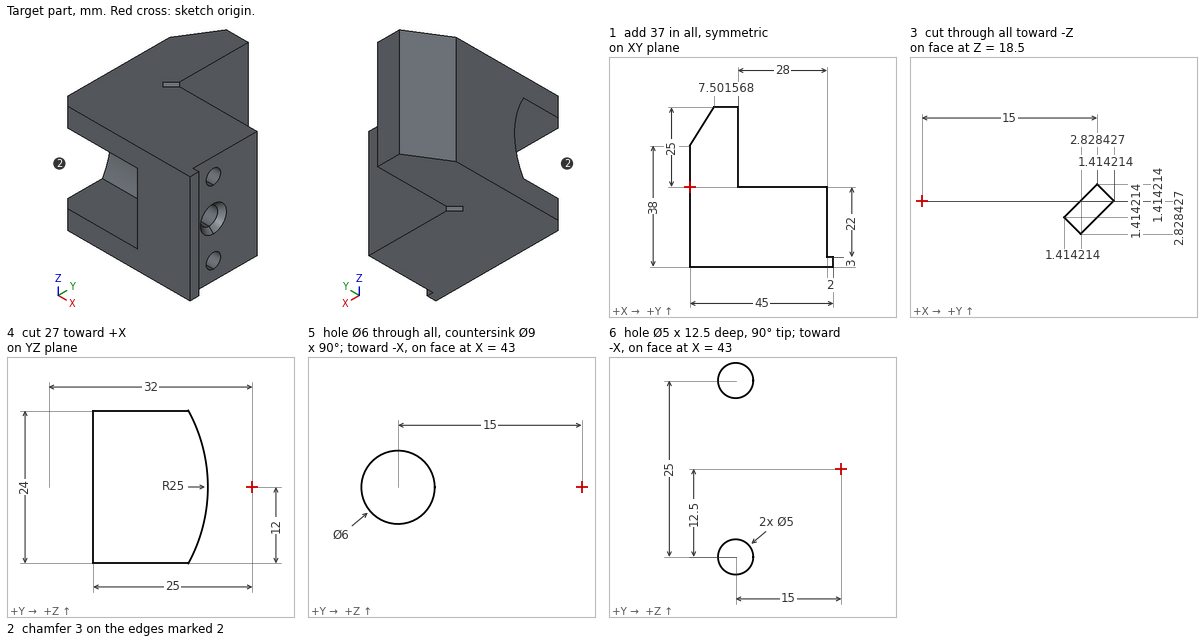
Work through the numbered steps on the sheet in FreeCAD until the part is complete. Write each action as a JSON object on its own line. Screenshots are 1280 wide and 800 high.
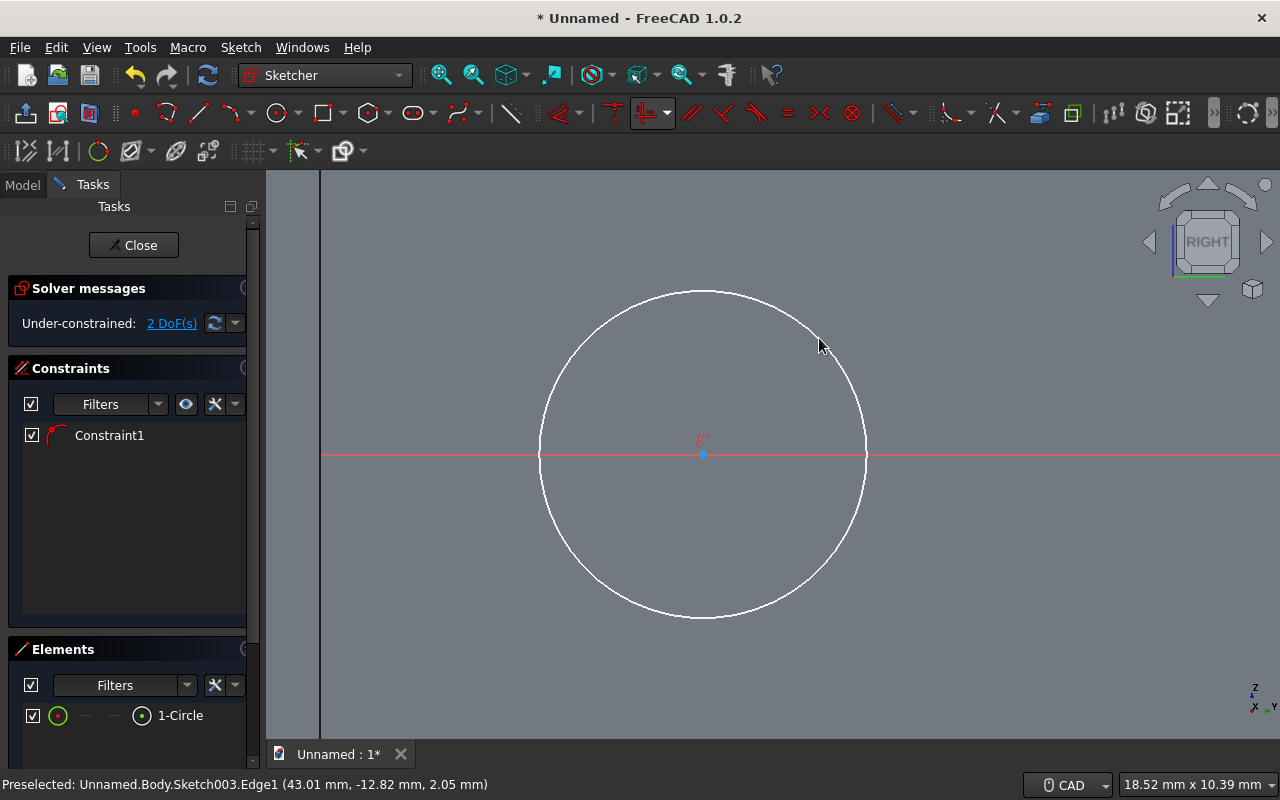
{"action": "key", "text": "d"}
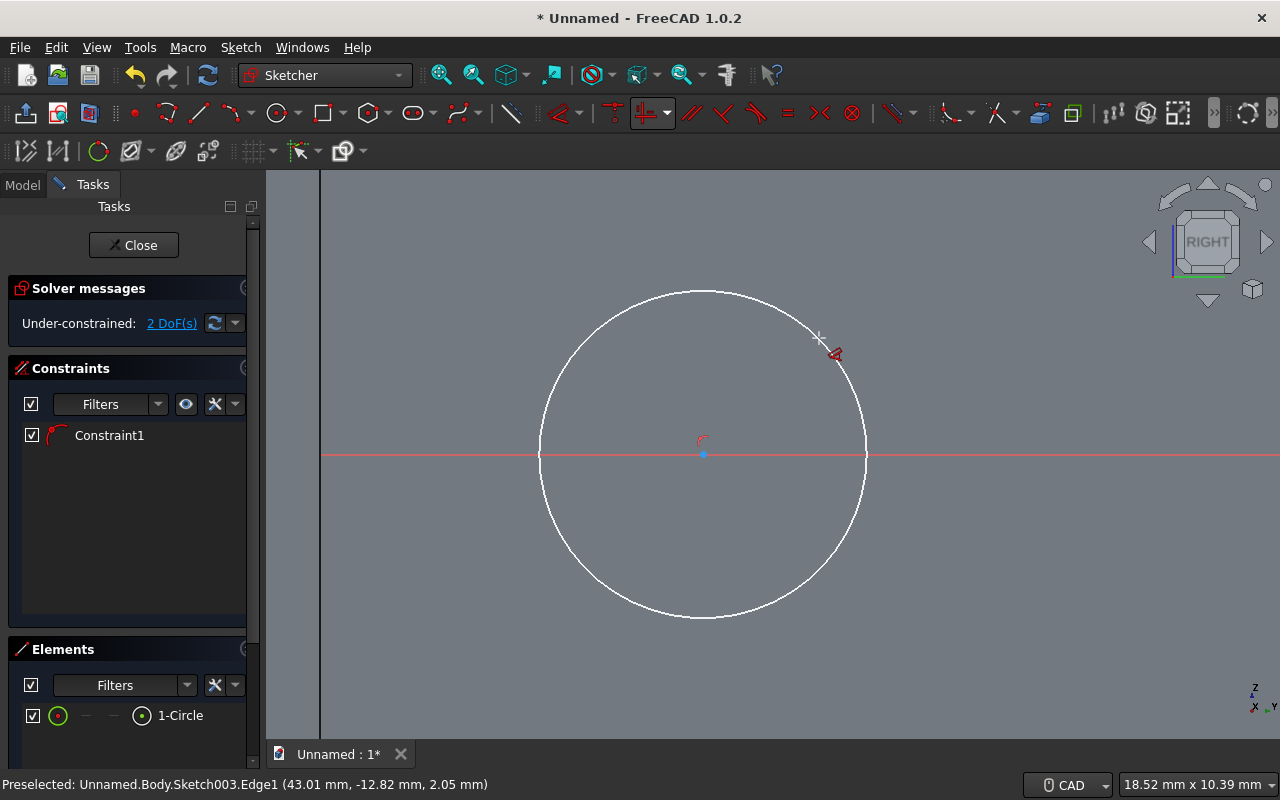
{"action": "left_click", "coordinate": [818, 338]}
{"action": "left_click", "coordinate": [840, 315]}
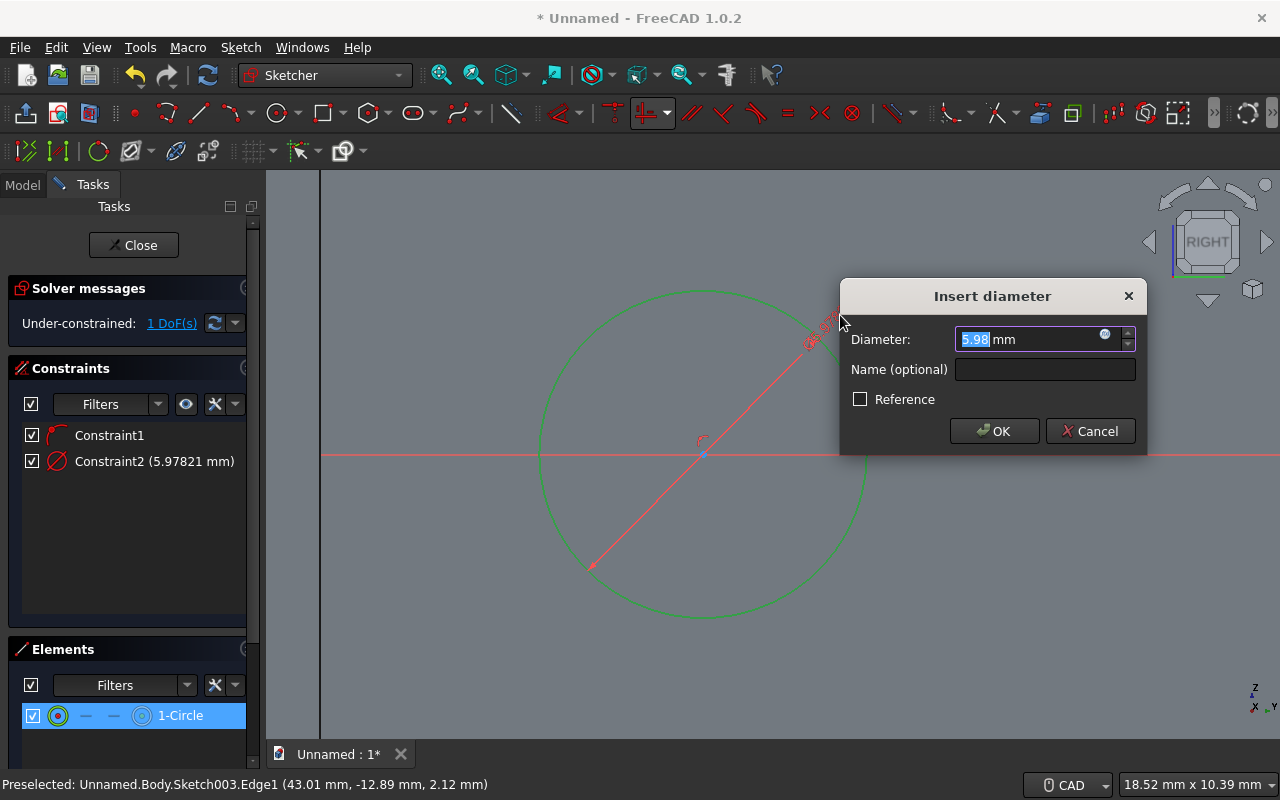
{"action": "type", "text": "6"}
{"action": "key", "text": "Return"}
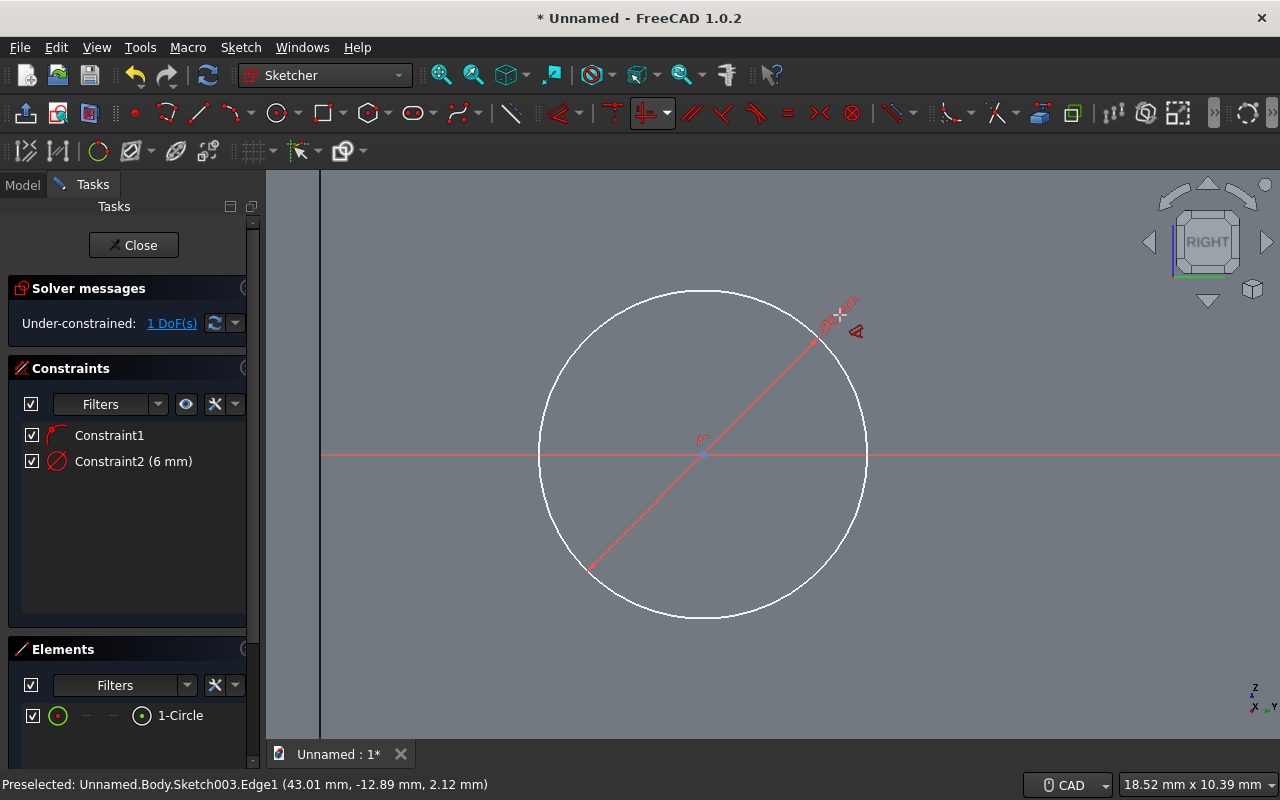
{"action": "left_click", "coordinate": [703, 454]}
{"action": "left_click", "coordinate": [909, 488]}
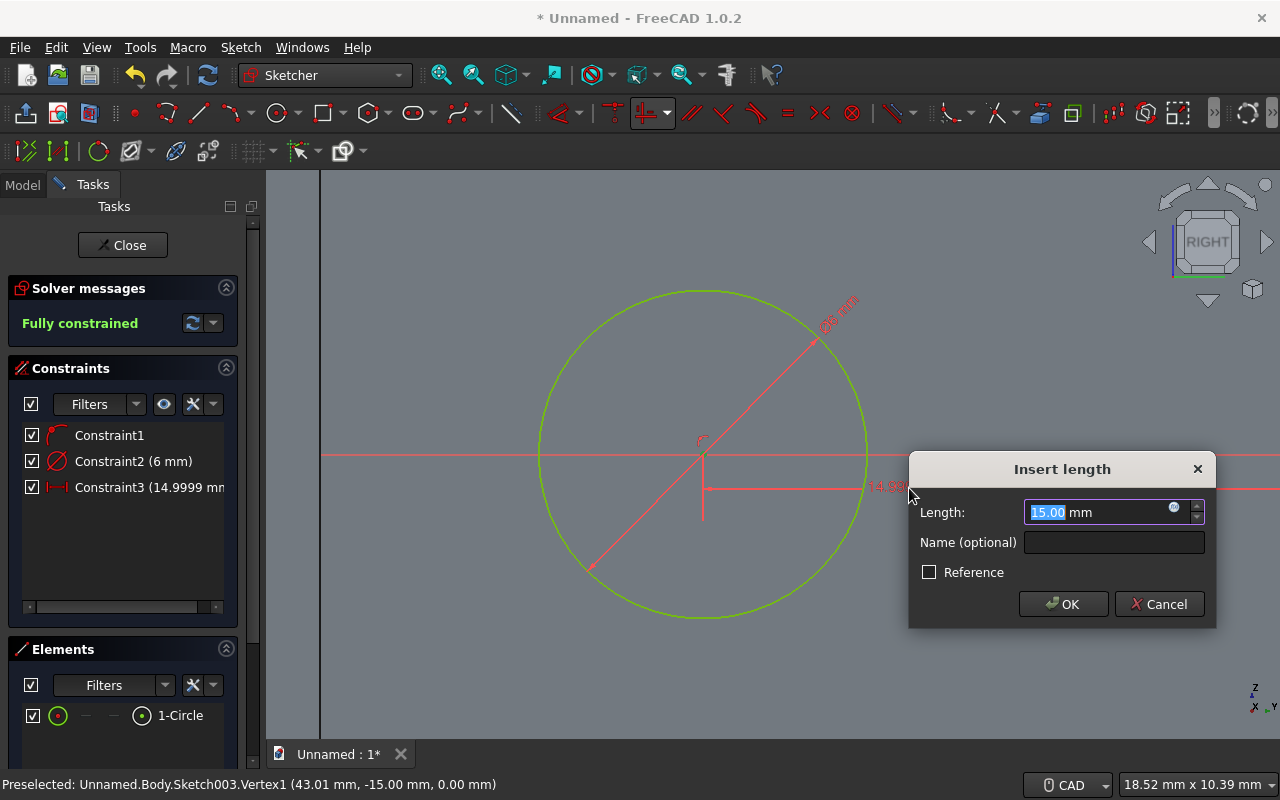
{"action": "type", "text": "15"}
{"action": "key", "text": "Return"}
{"action": "key", "text": "Escape"}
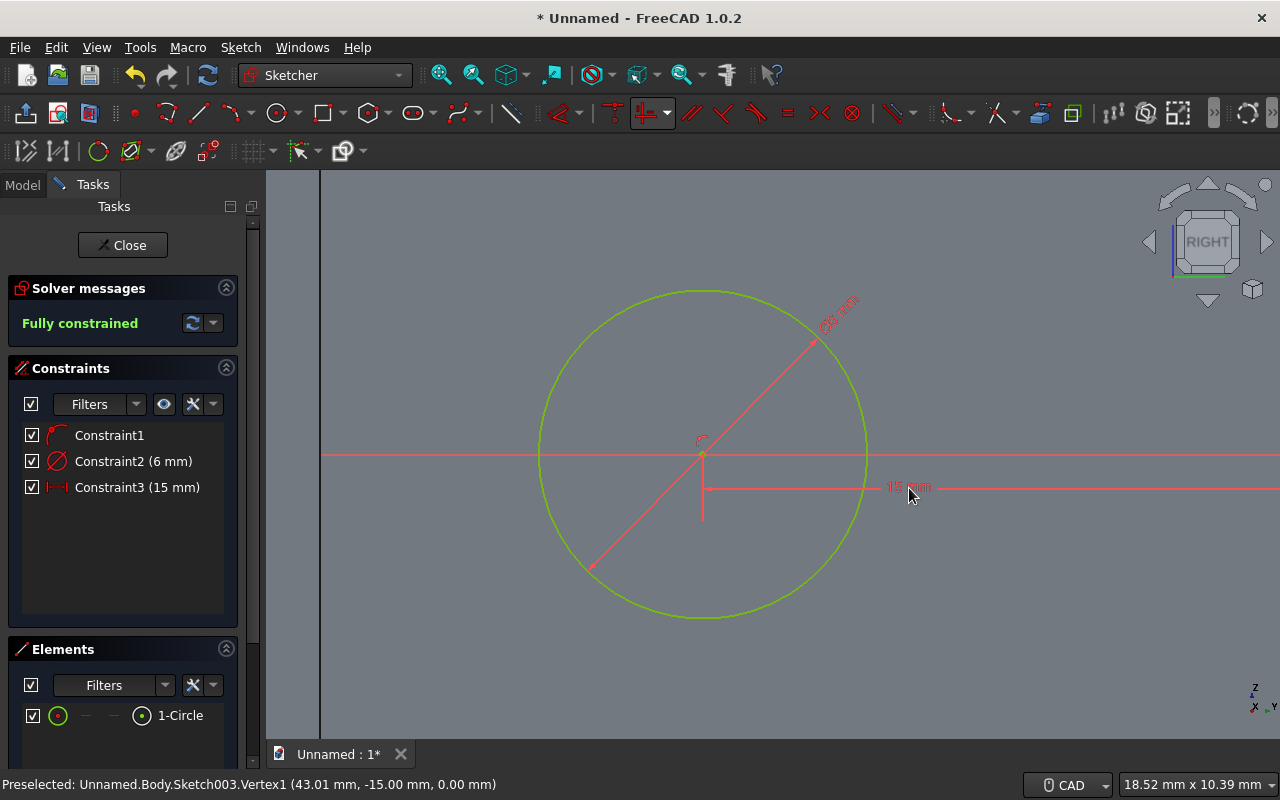
{"action": "left_click", "coordinate": [123, 245]}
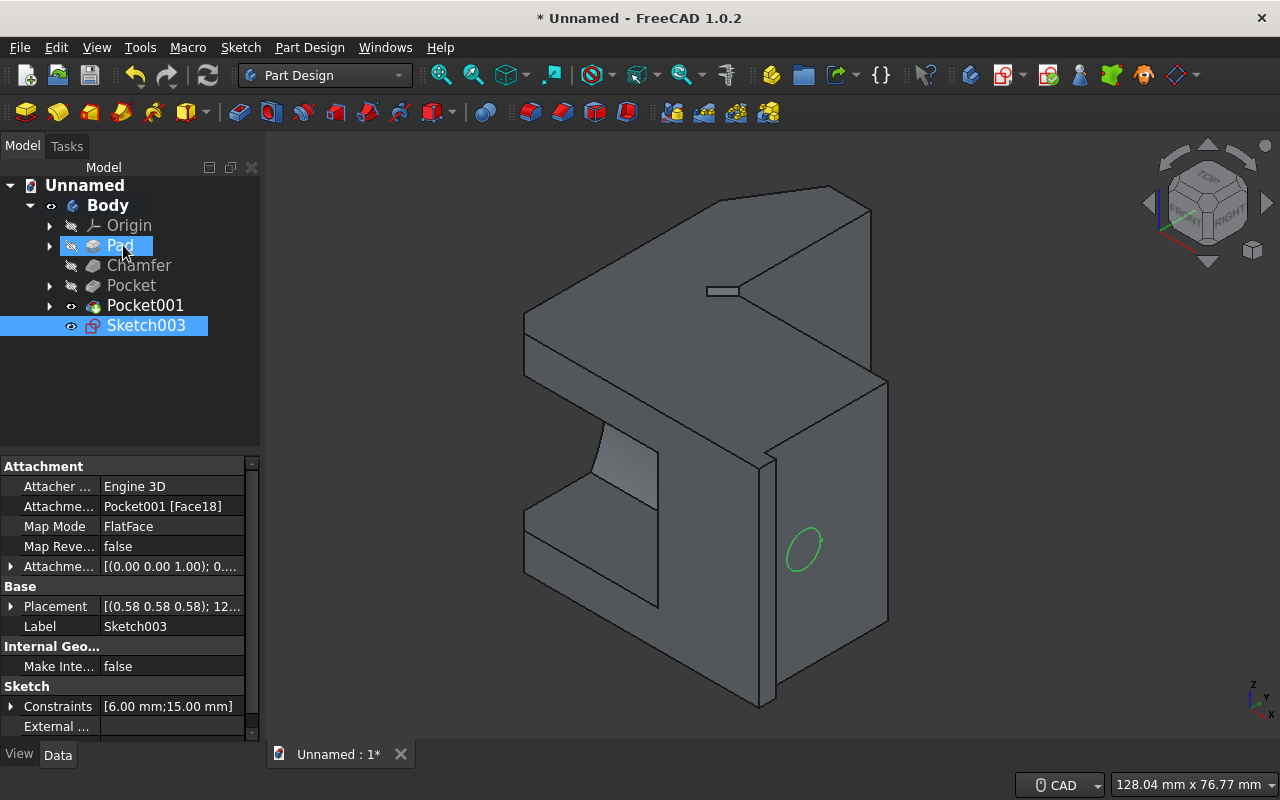
{"action": "left_click", "coordinate": [272, 112]}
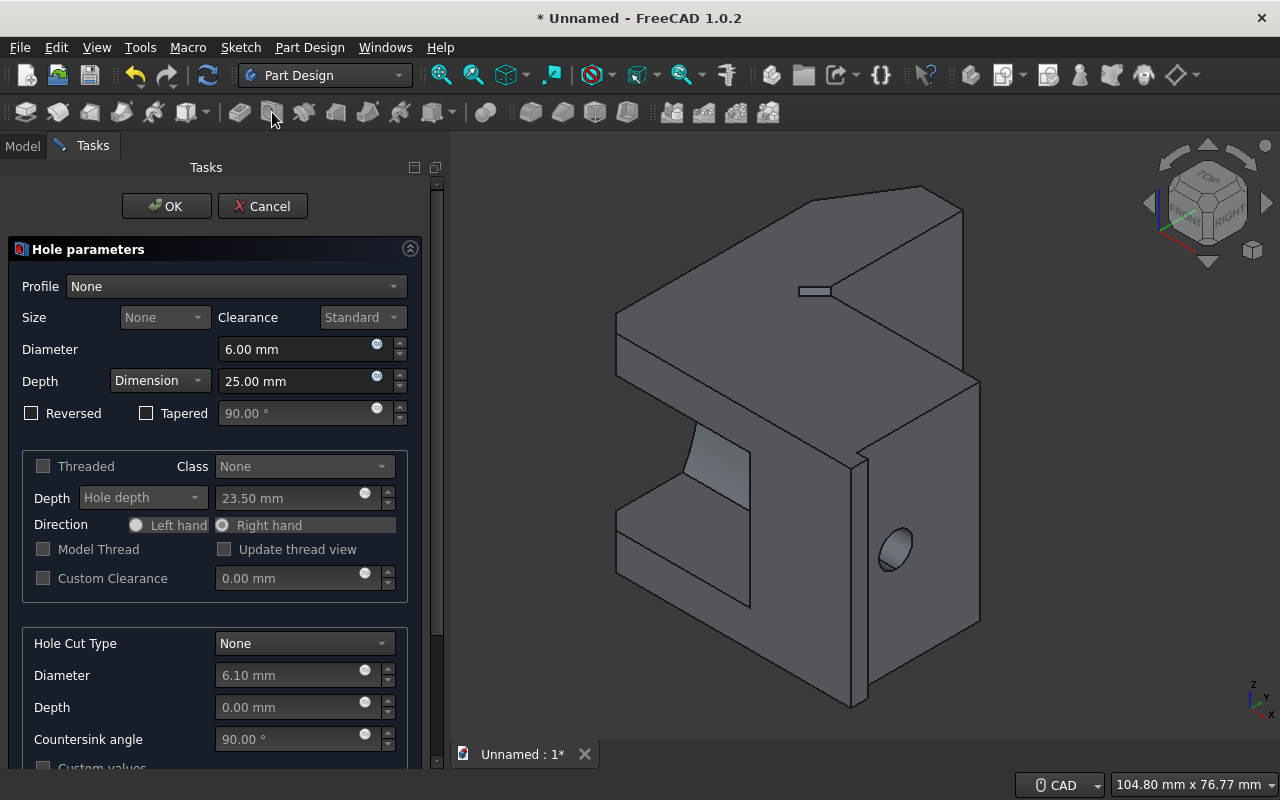
{"action": "triple_click", "coordinate": [305, 349]}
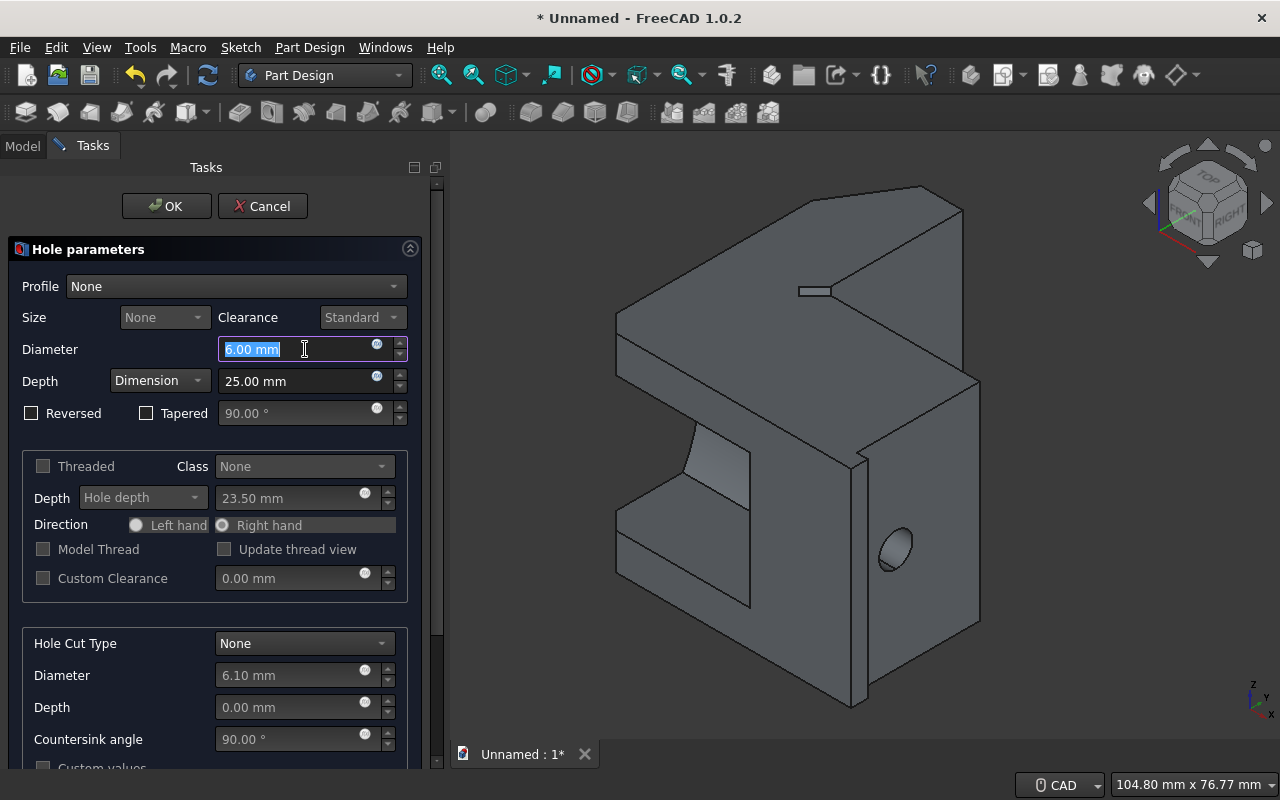
{"action": "type", "text": "6"}
{"action": "key", "text": "Tab"}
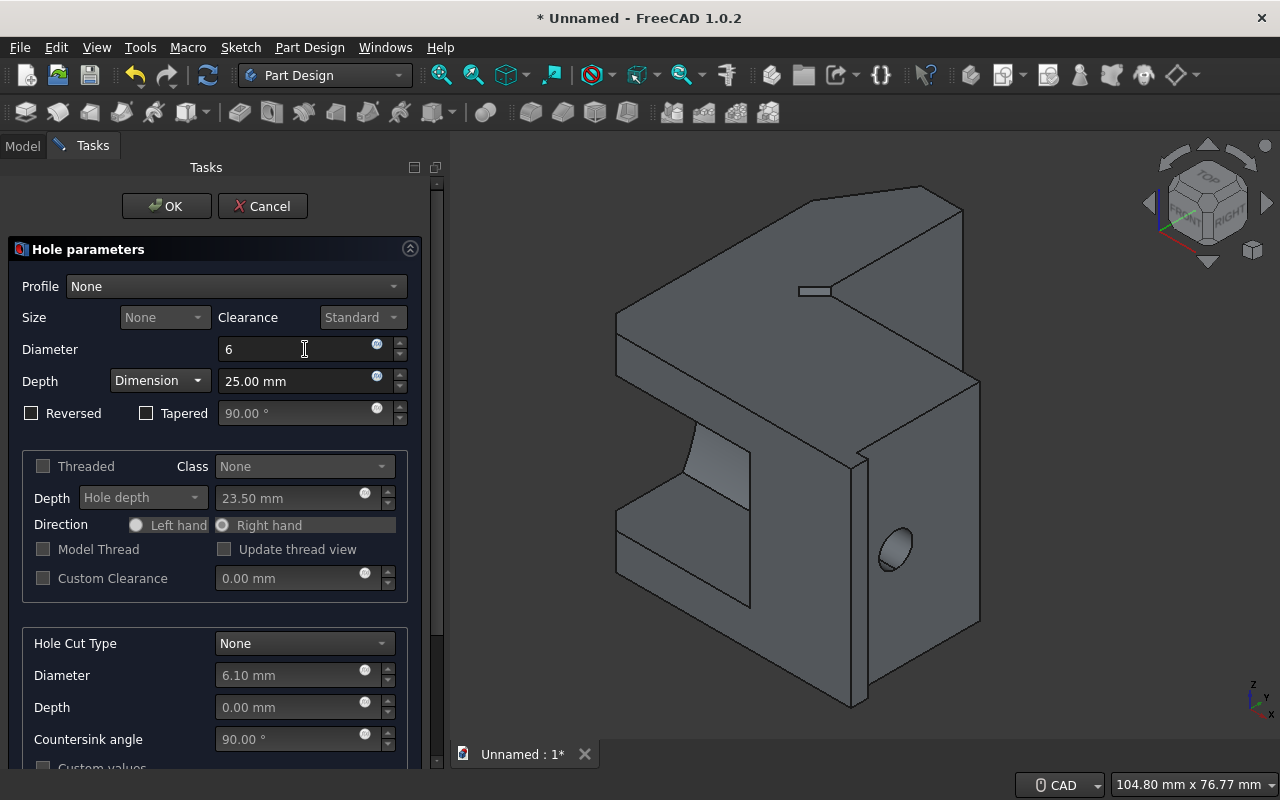
{"action": "left_click", "coordinate": [161, 380]}